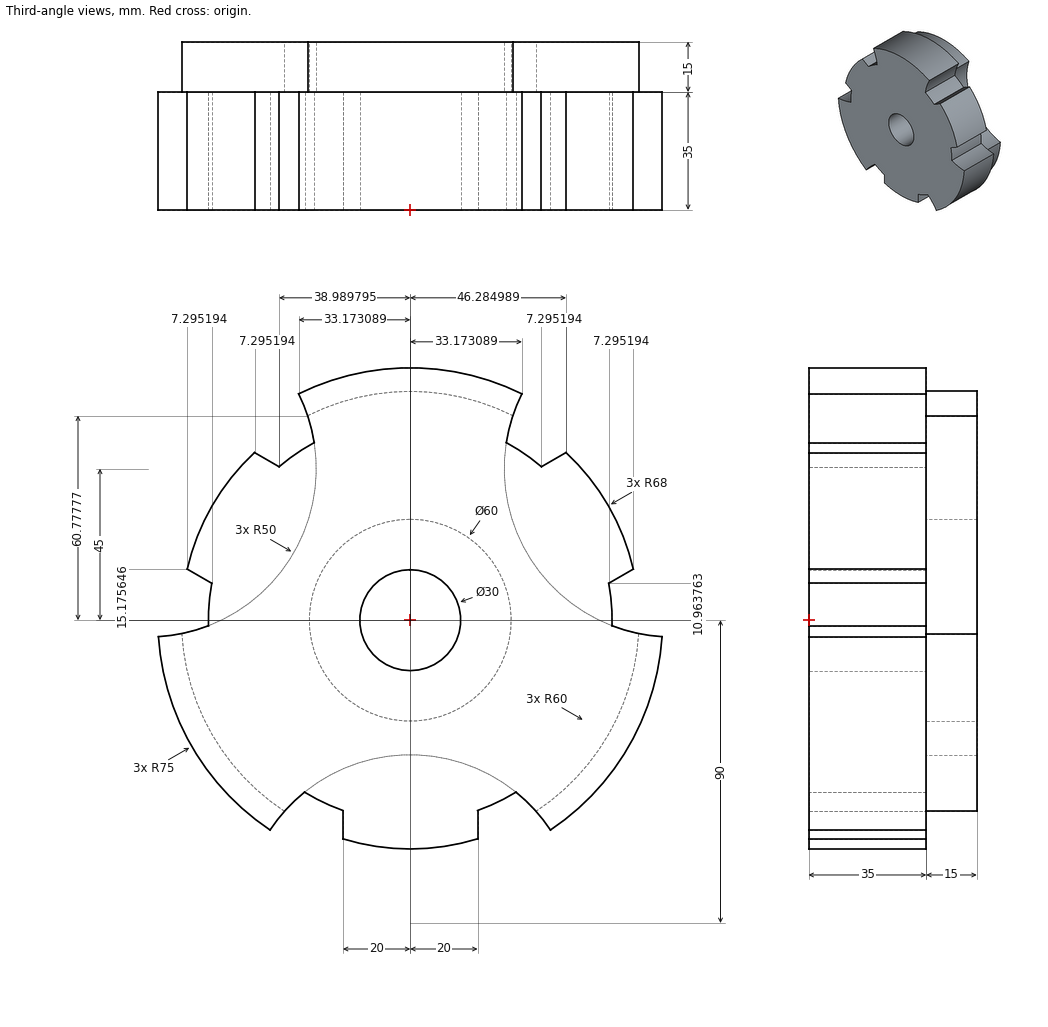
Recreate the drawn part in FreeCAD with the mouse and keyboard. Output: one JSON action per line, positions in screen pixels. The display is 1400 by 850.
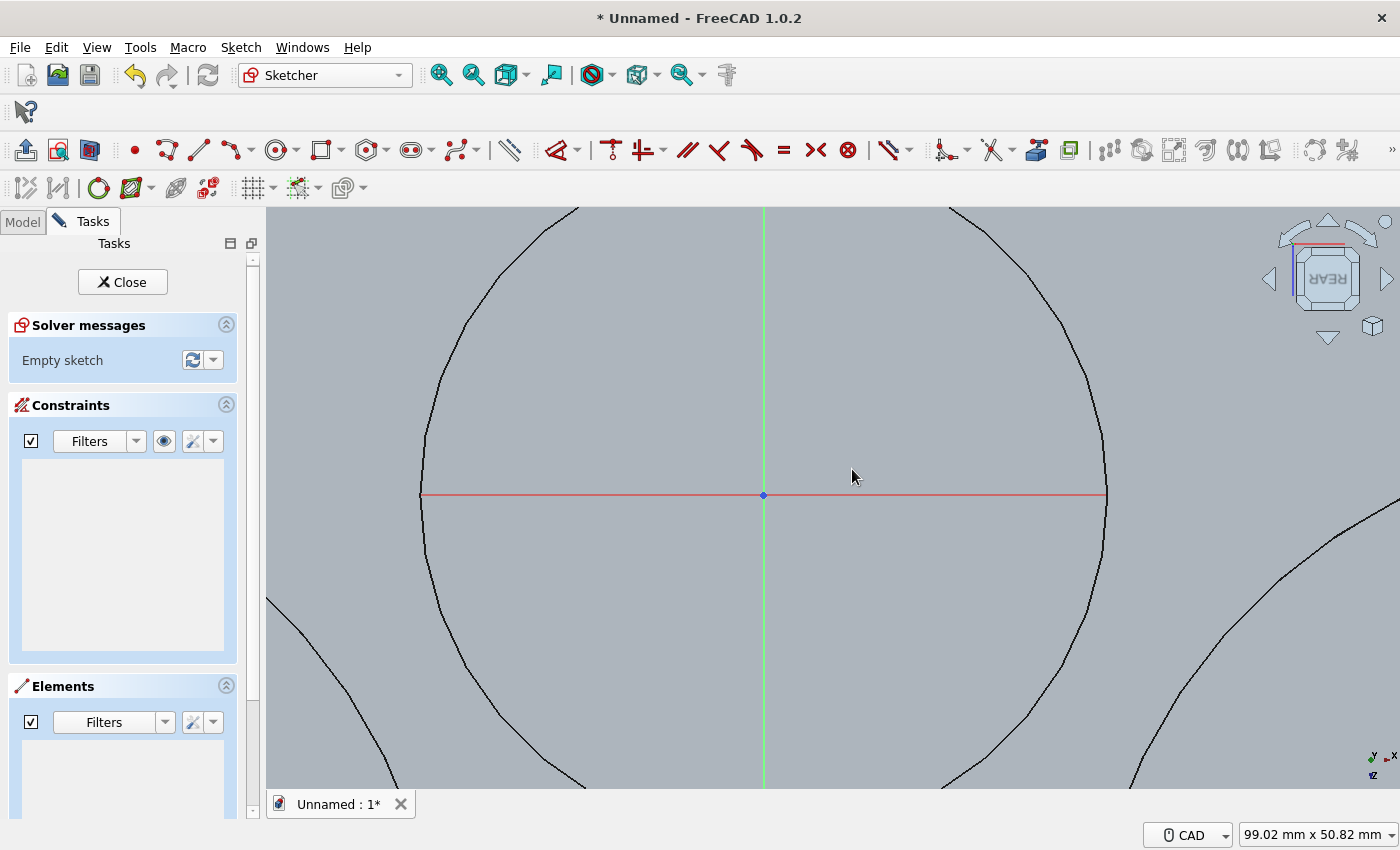
{"action": "left_click", "coordinate": [276, 150]}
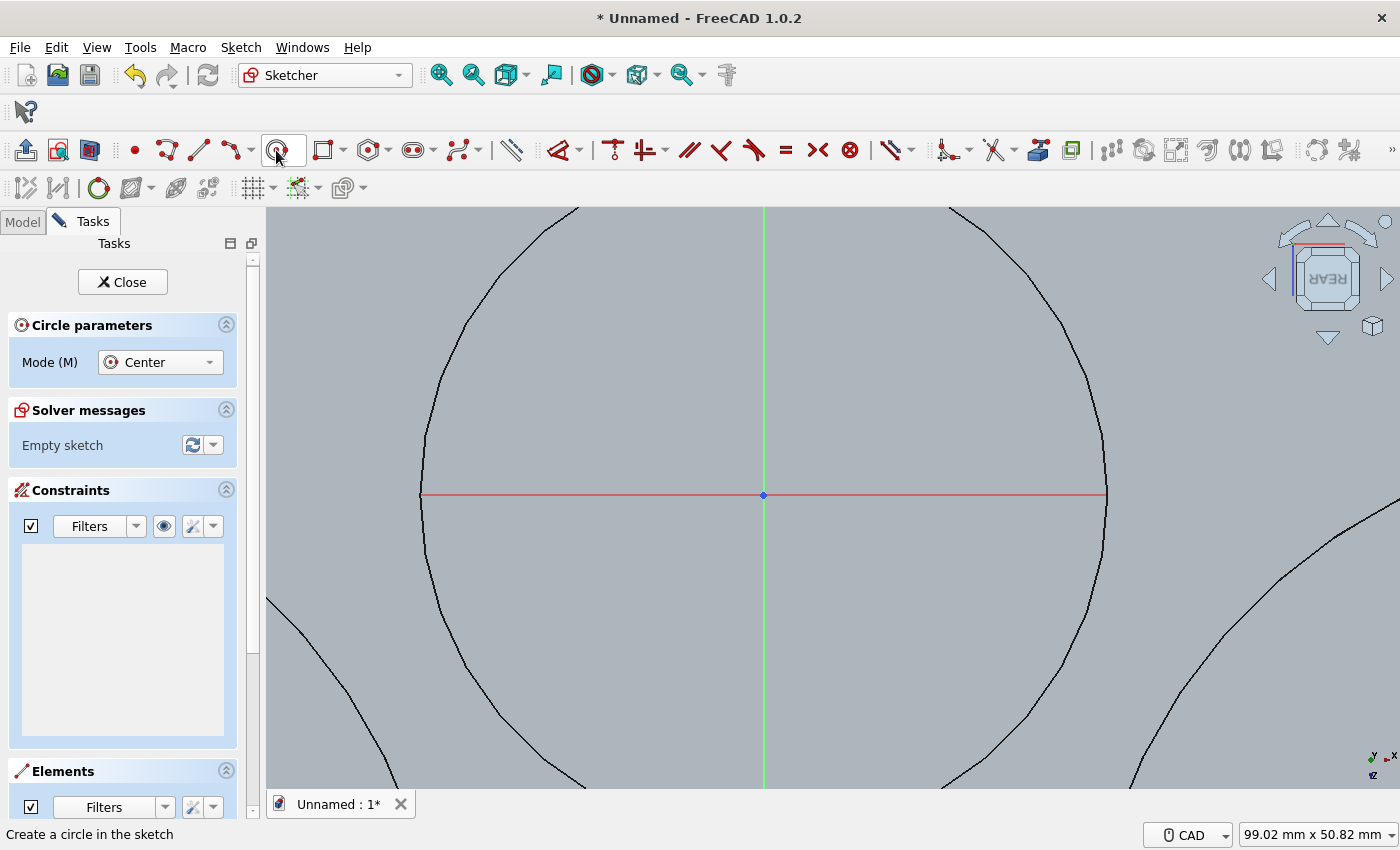
{"action": "left_click", "coordinate": [764, 495]}
{"action": "left_click", "coordinate": [885, 374]}
{"action": "key", "text": "Escape"}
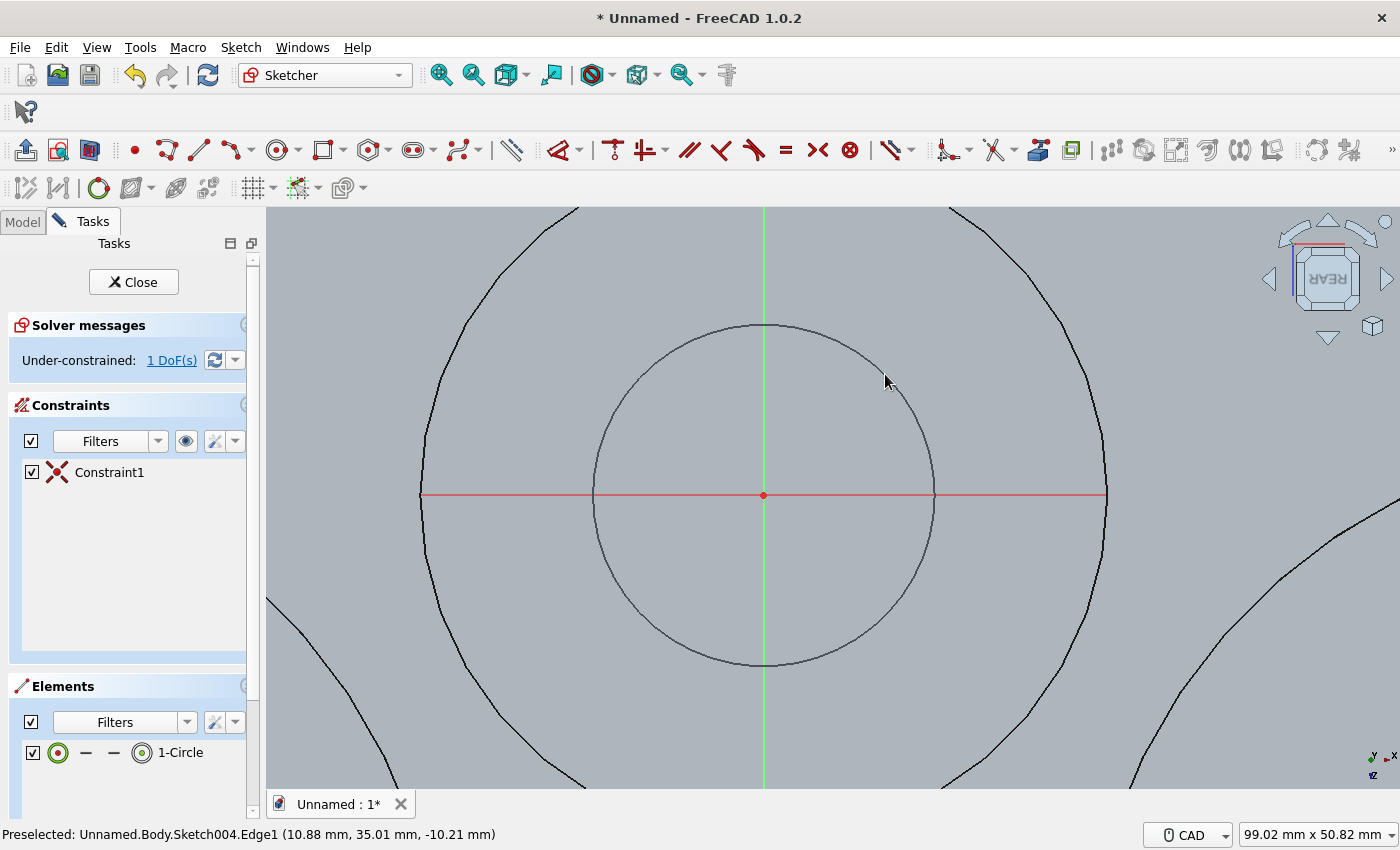
{"action": "left_click", "coordinate": [558, 150]}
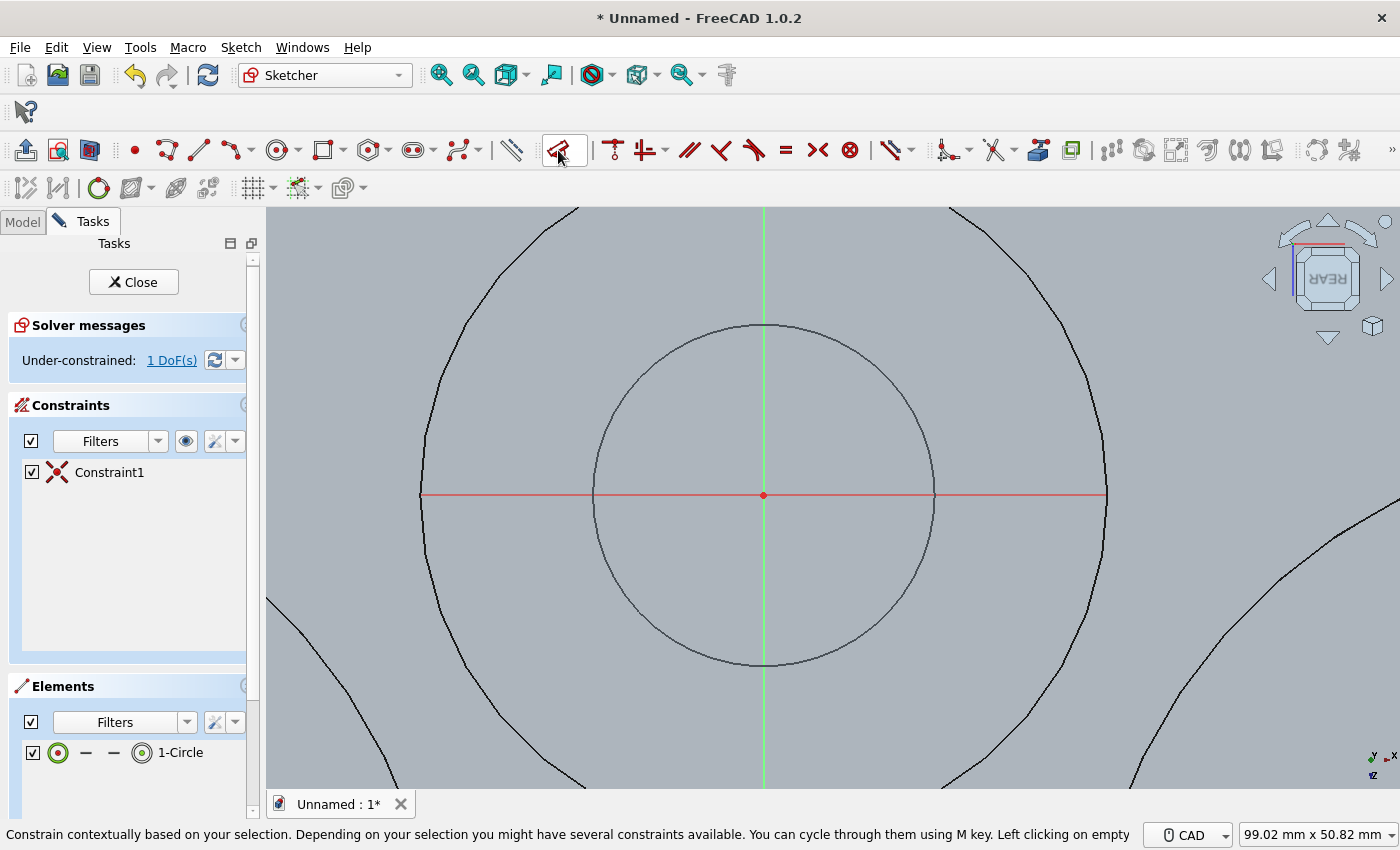
{"action": "left_click", "coordinate": [884, 374]}
{"action": "left_click", "coordinate": [907, 351]}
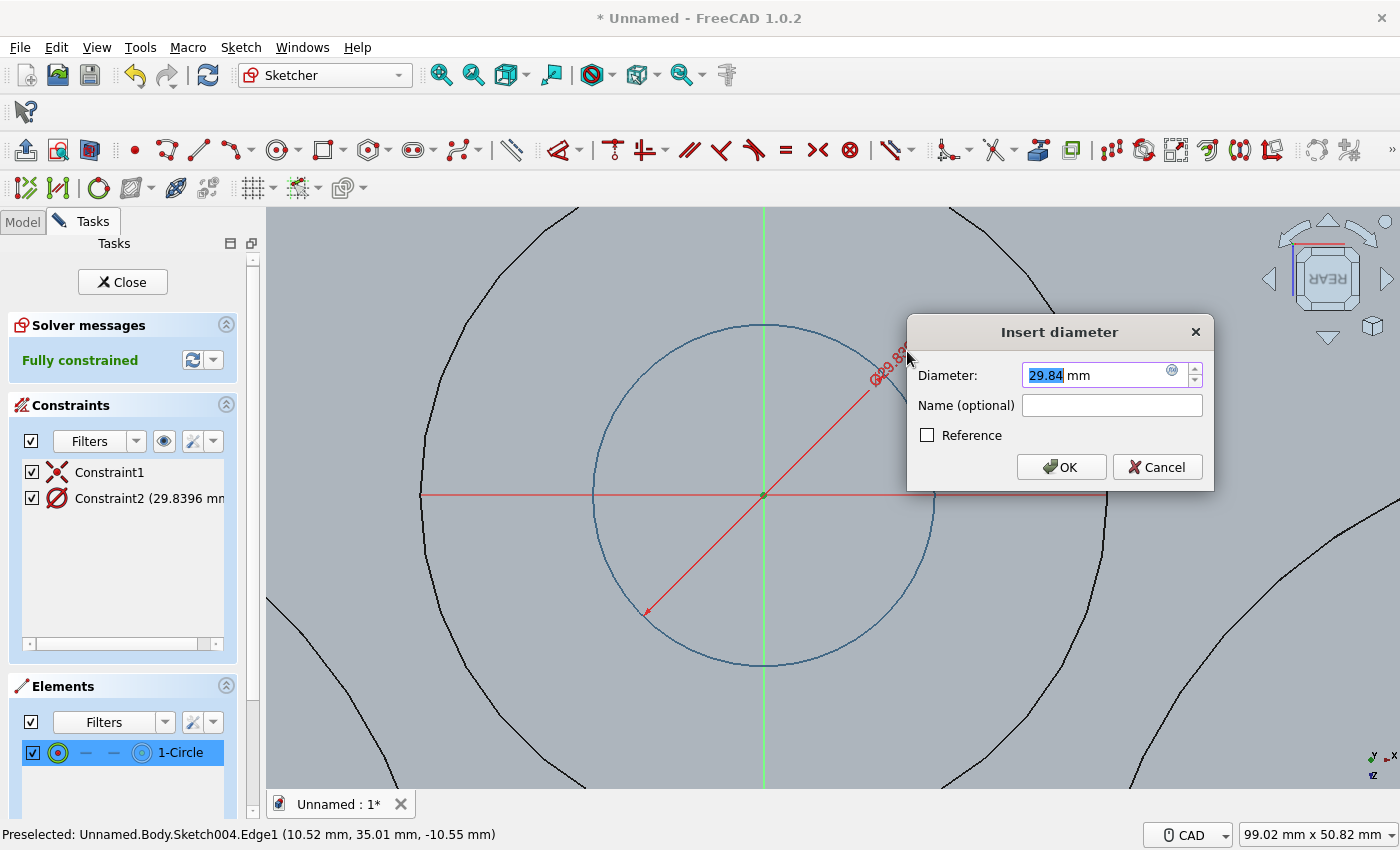
{"action": "type", "text": "30"}
{"action": "key", "text": "Return"}
{"action": "key", "text": "Escape"}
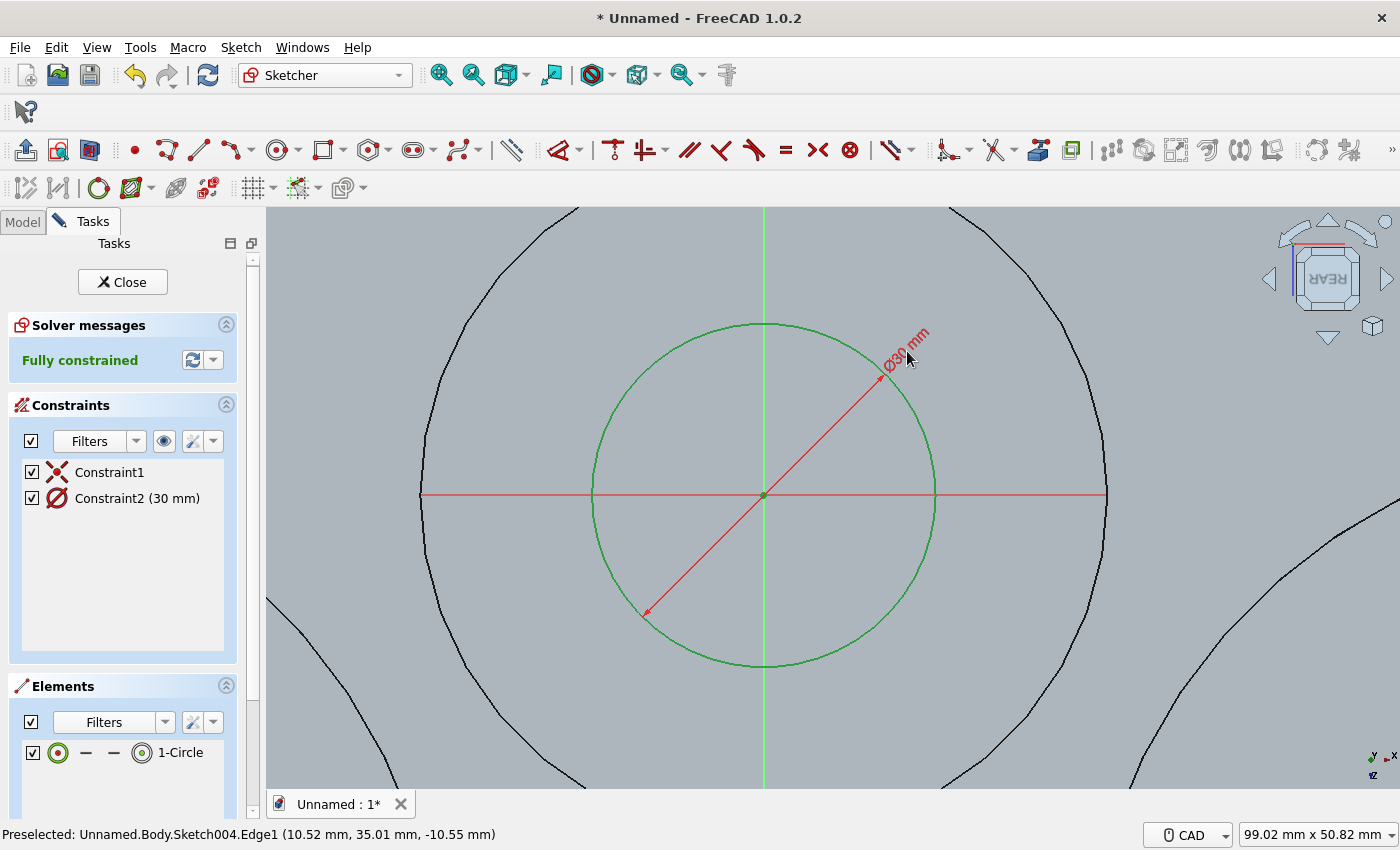
{"action": "left_click", "coordinate": [123, 282]}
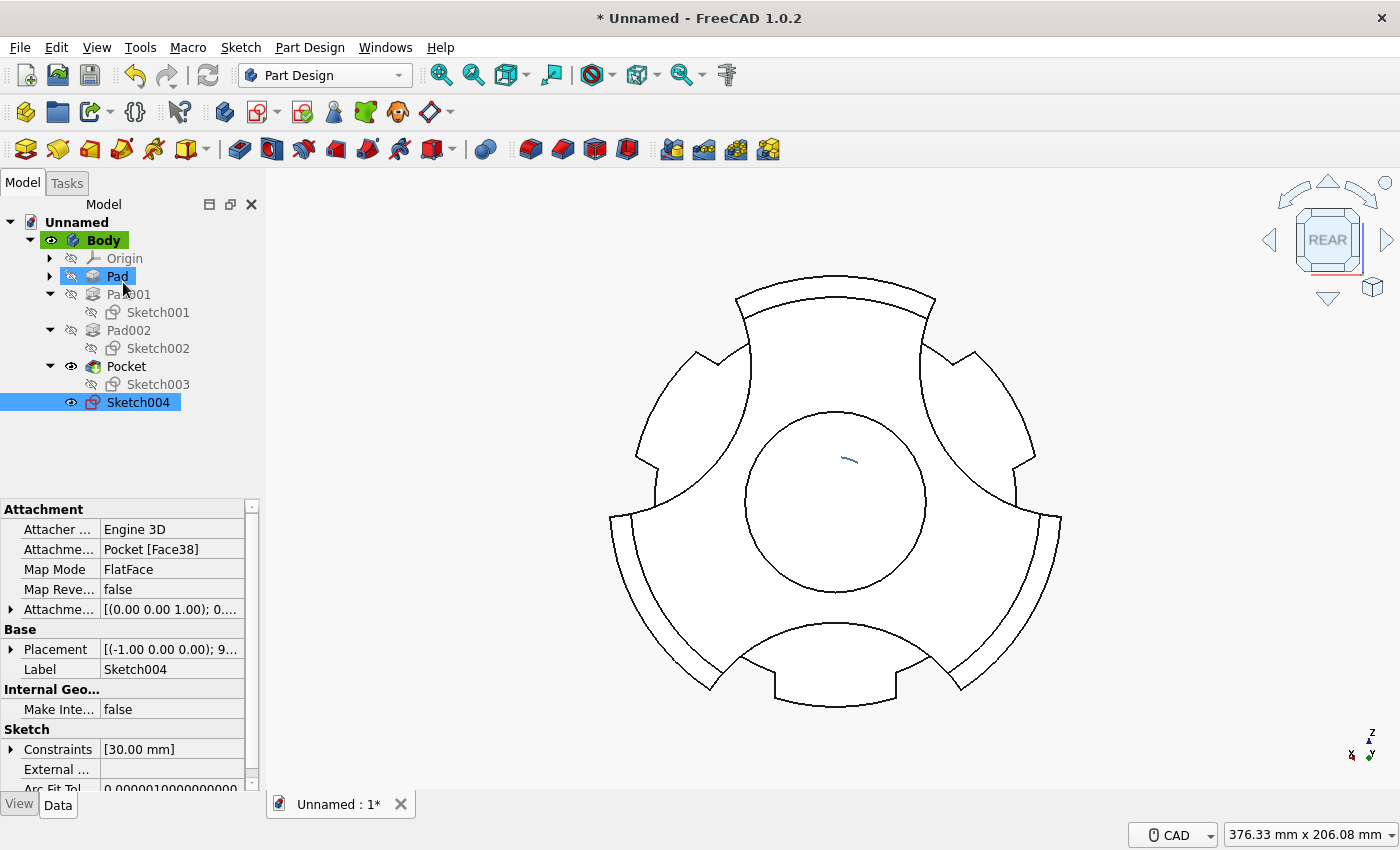
{"action": "left_click", "coordinate": [240, 150]}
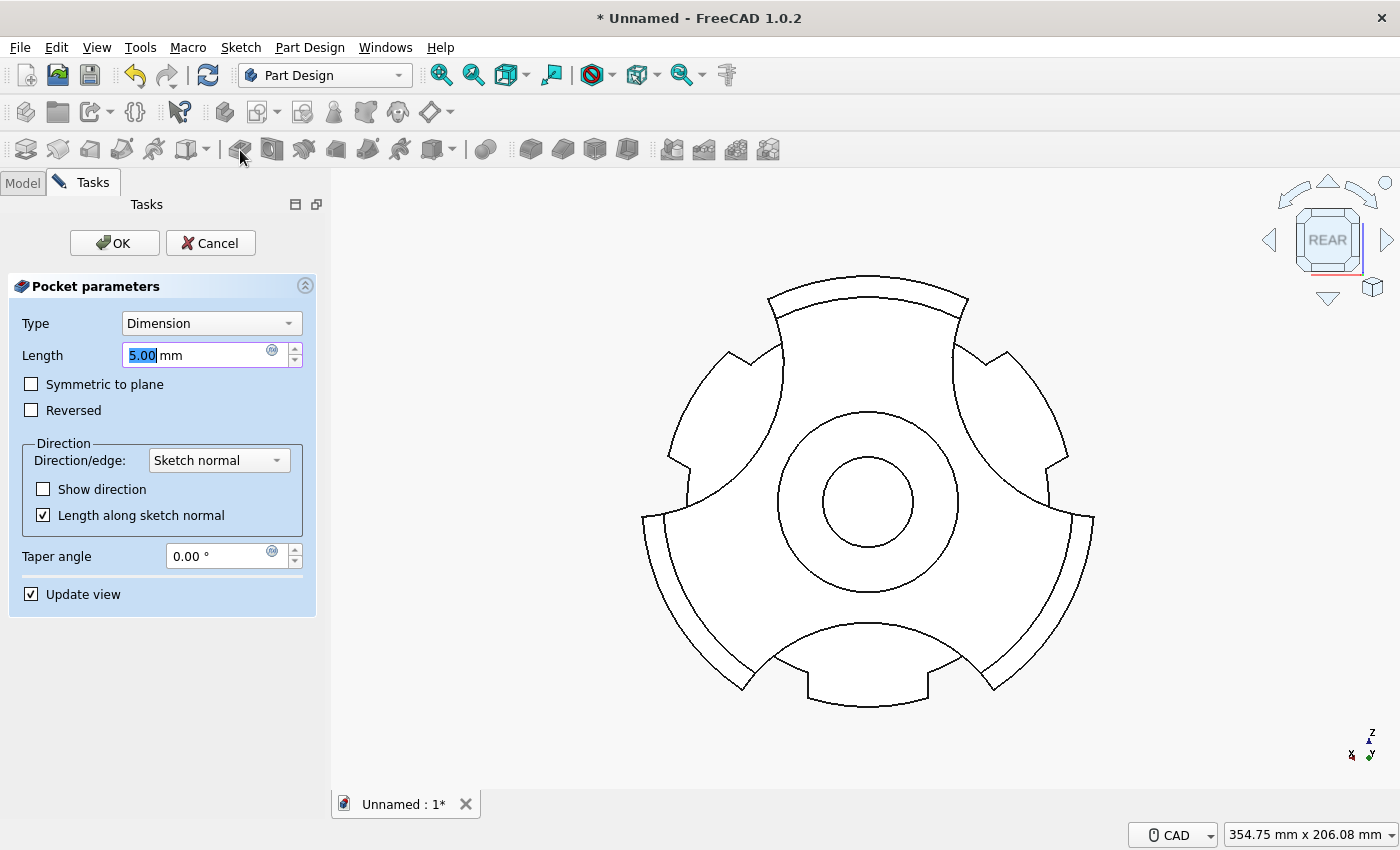
{"action": "type", "text": "35"}
{"action": "key", "text": "Tab"}